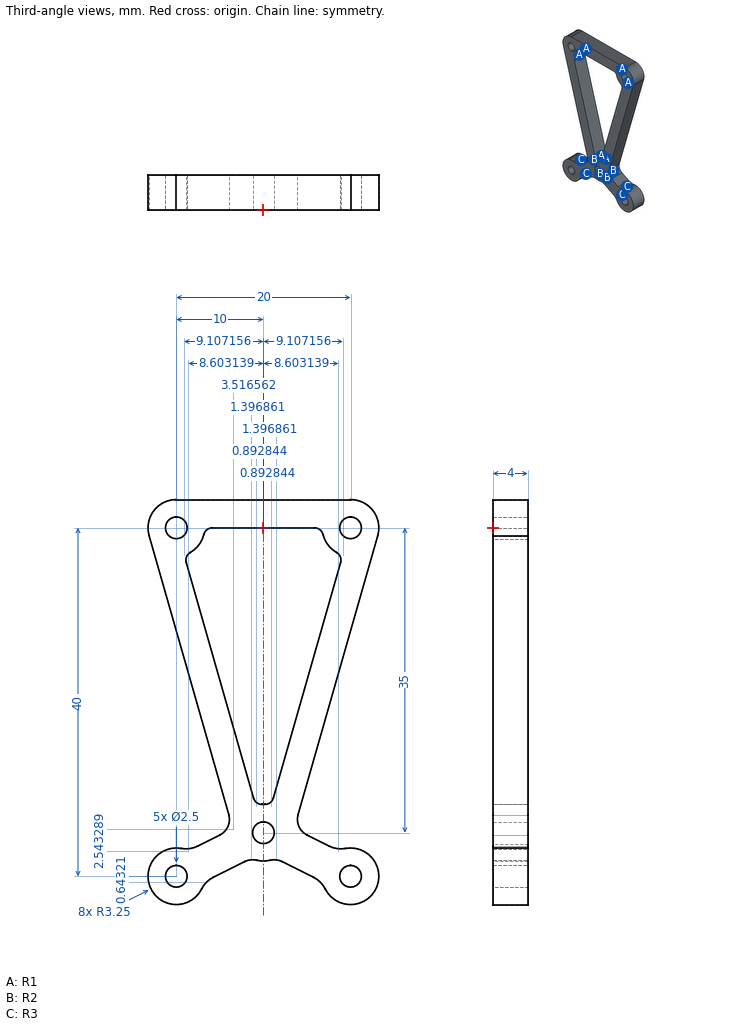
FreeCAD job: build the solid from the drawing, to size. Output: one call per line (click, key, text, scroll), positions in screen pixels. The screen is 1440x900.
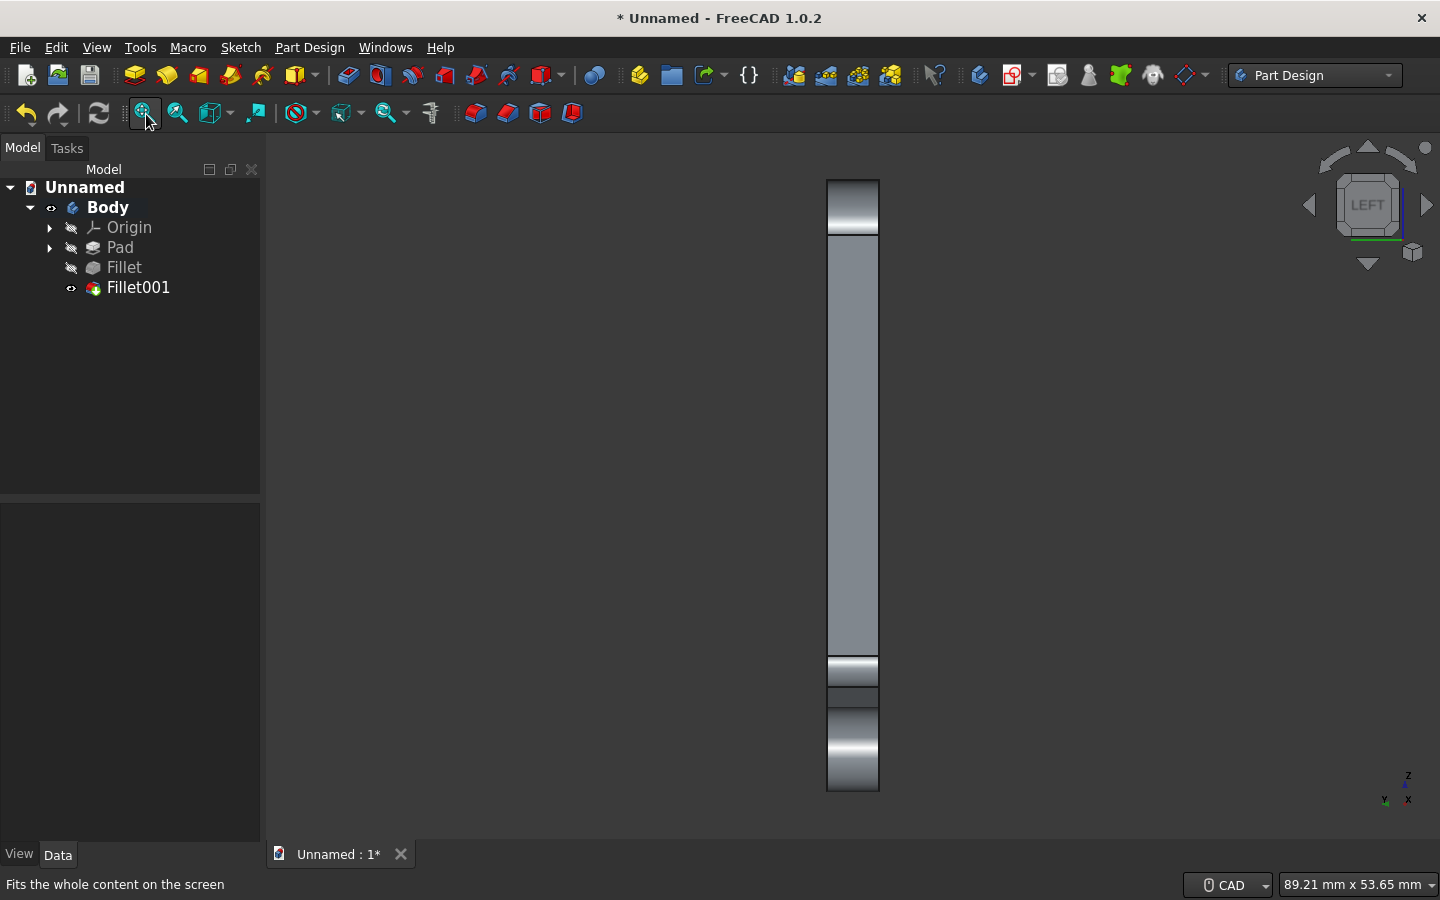
key(v)
key(3)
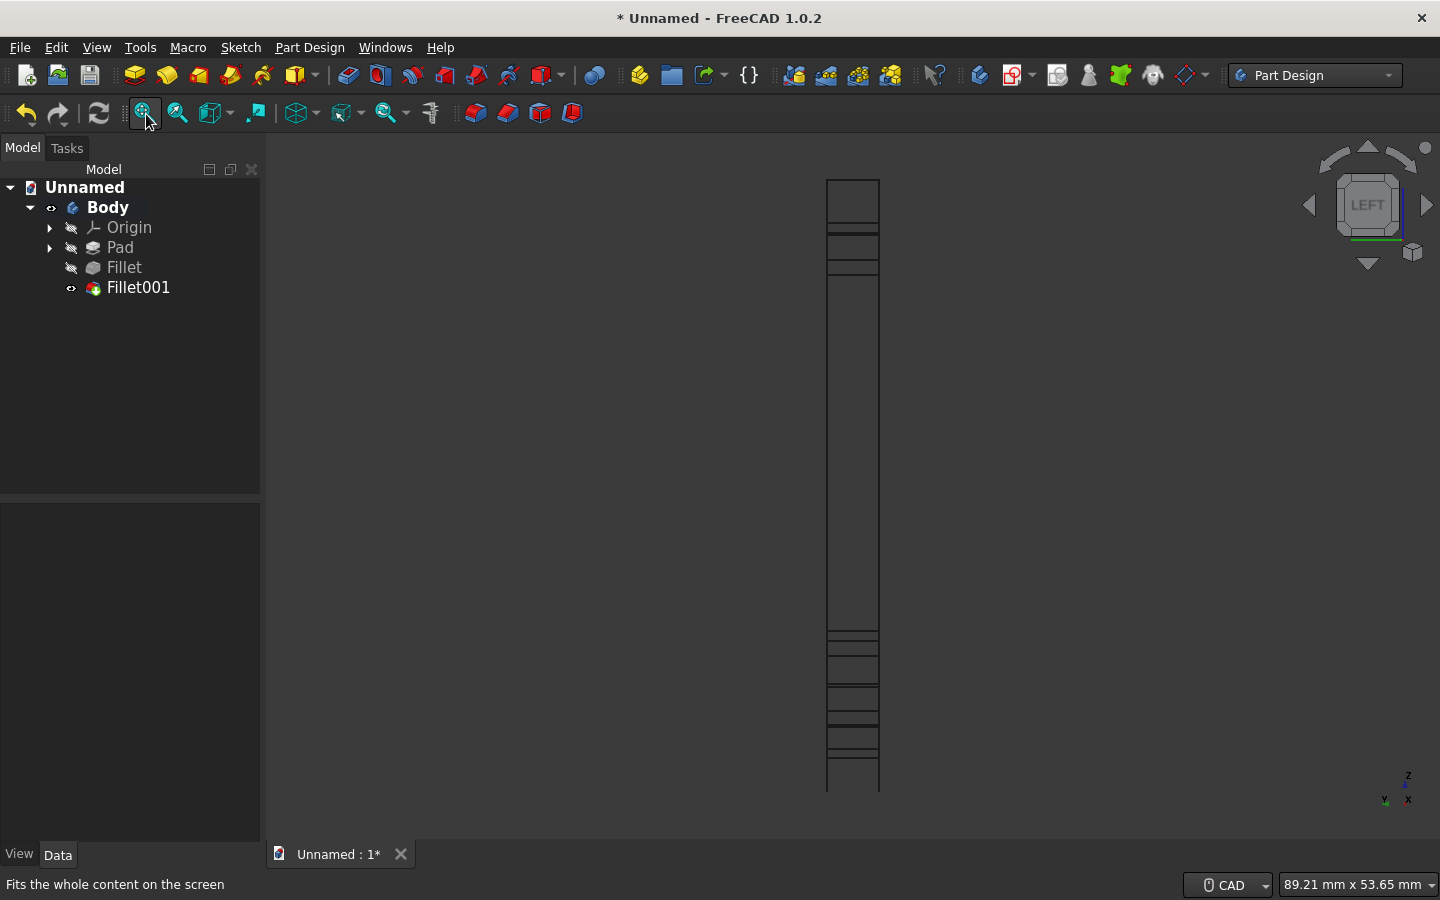
key(0)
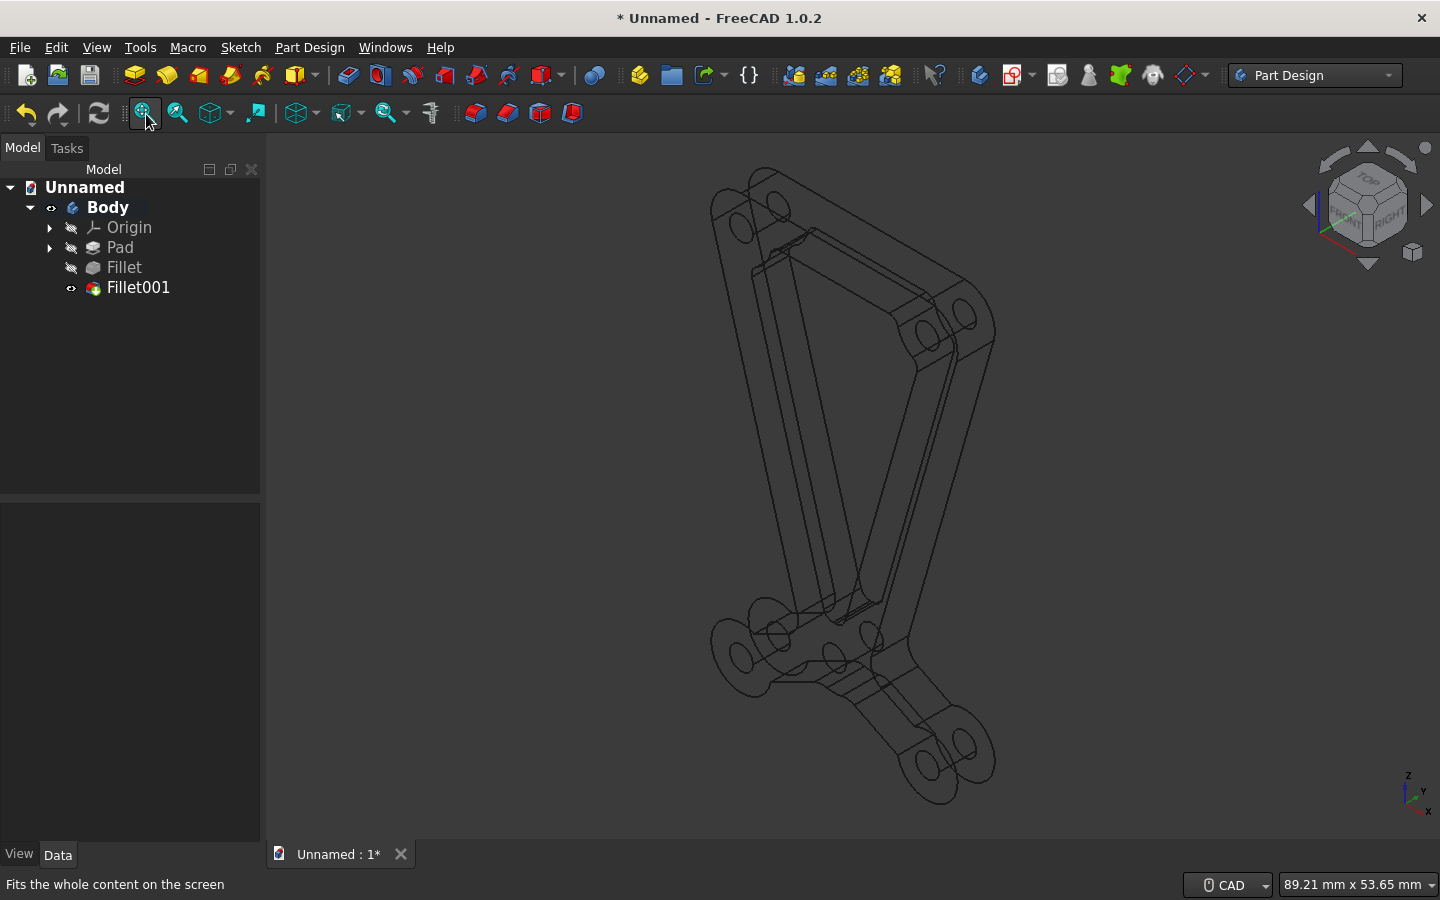
click(773, 622)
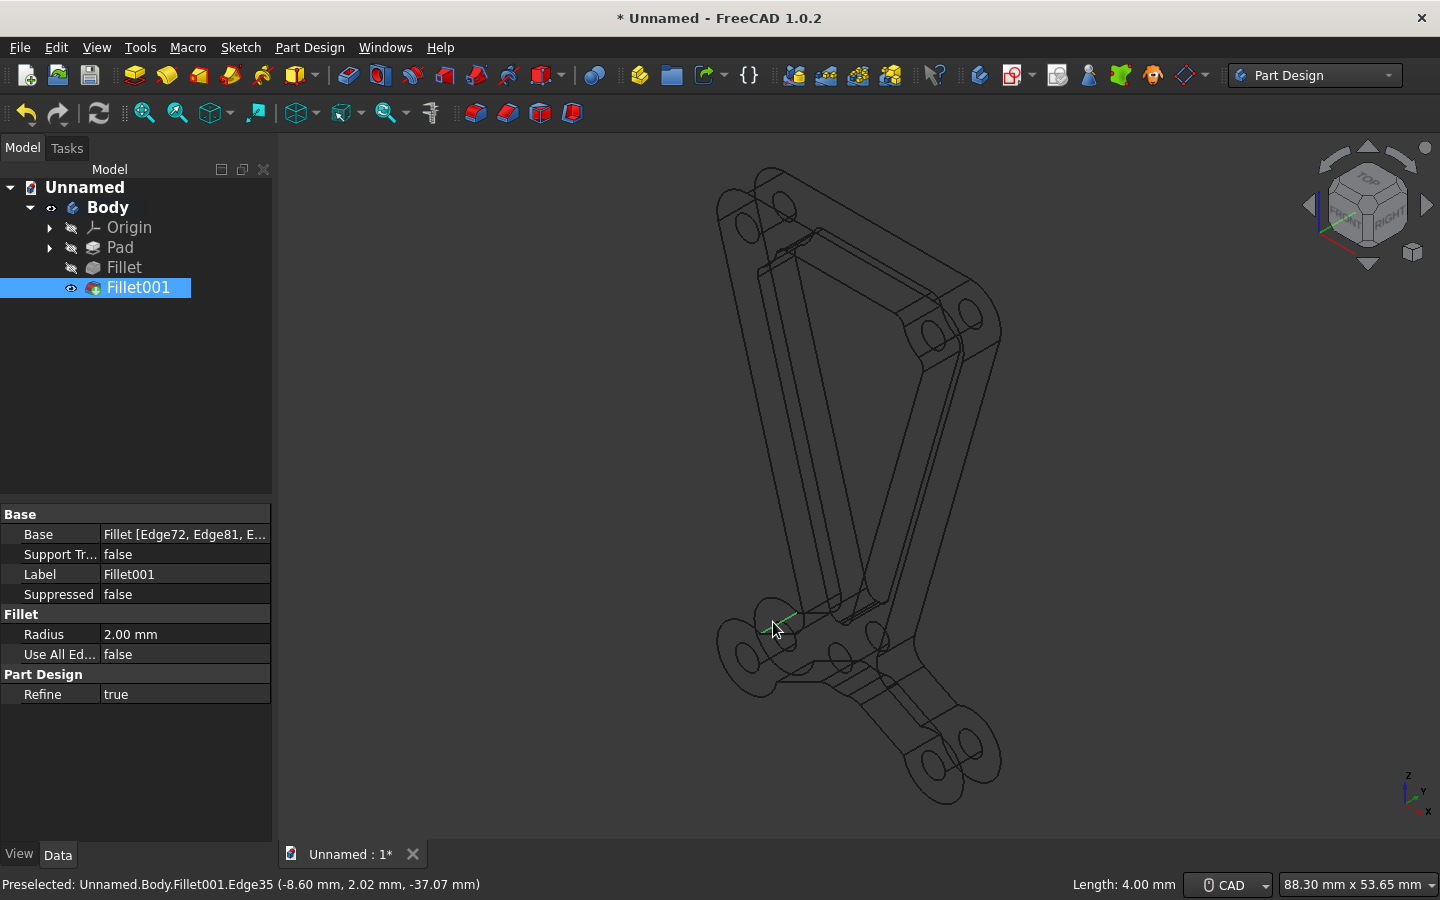
click(796, 670, ctrl)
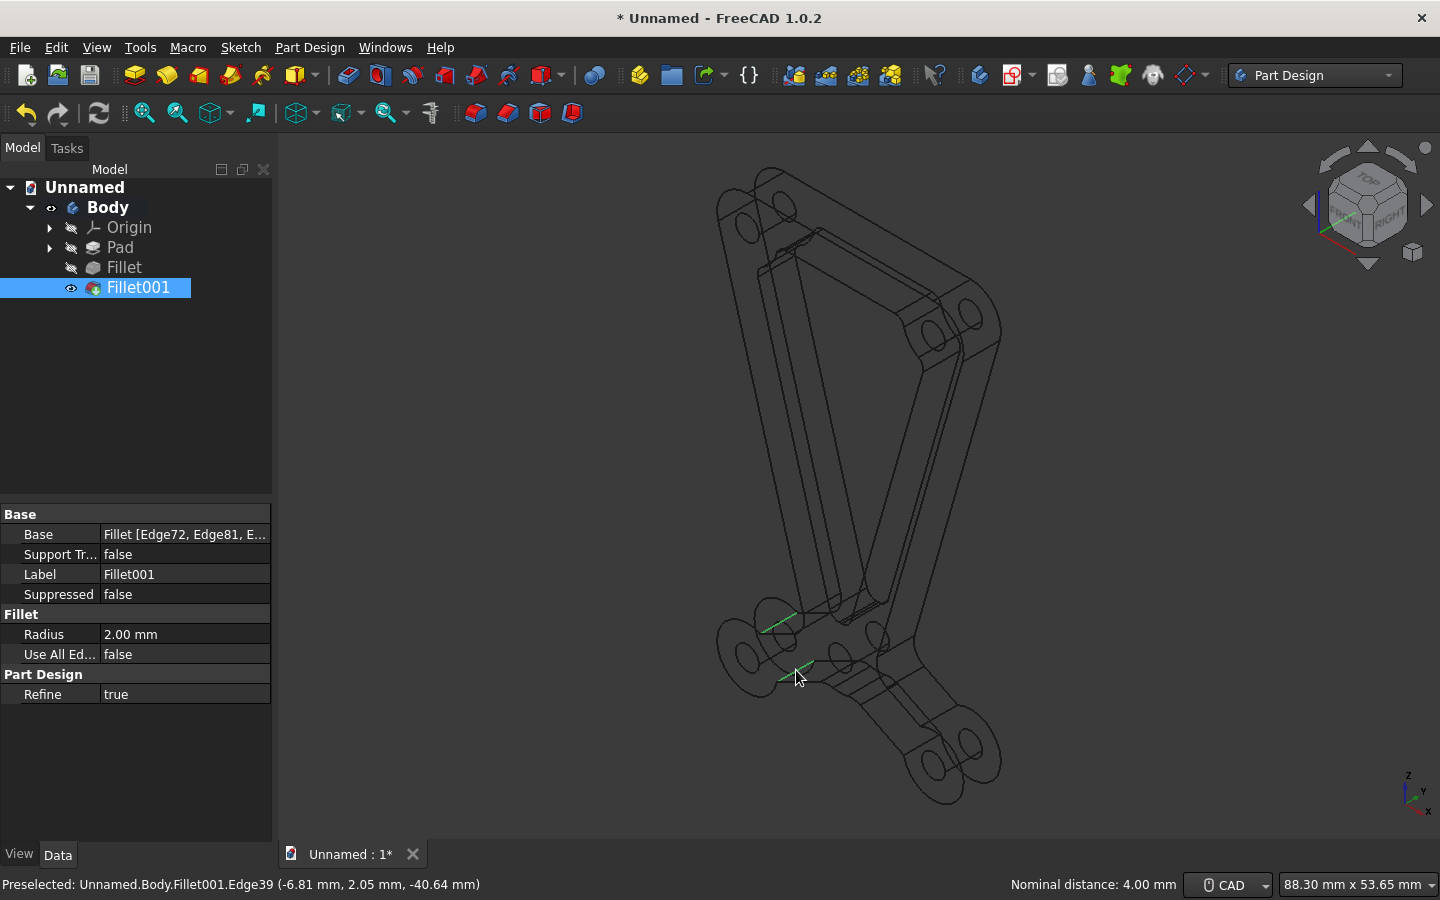
click(922, 744, ctrl)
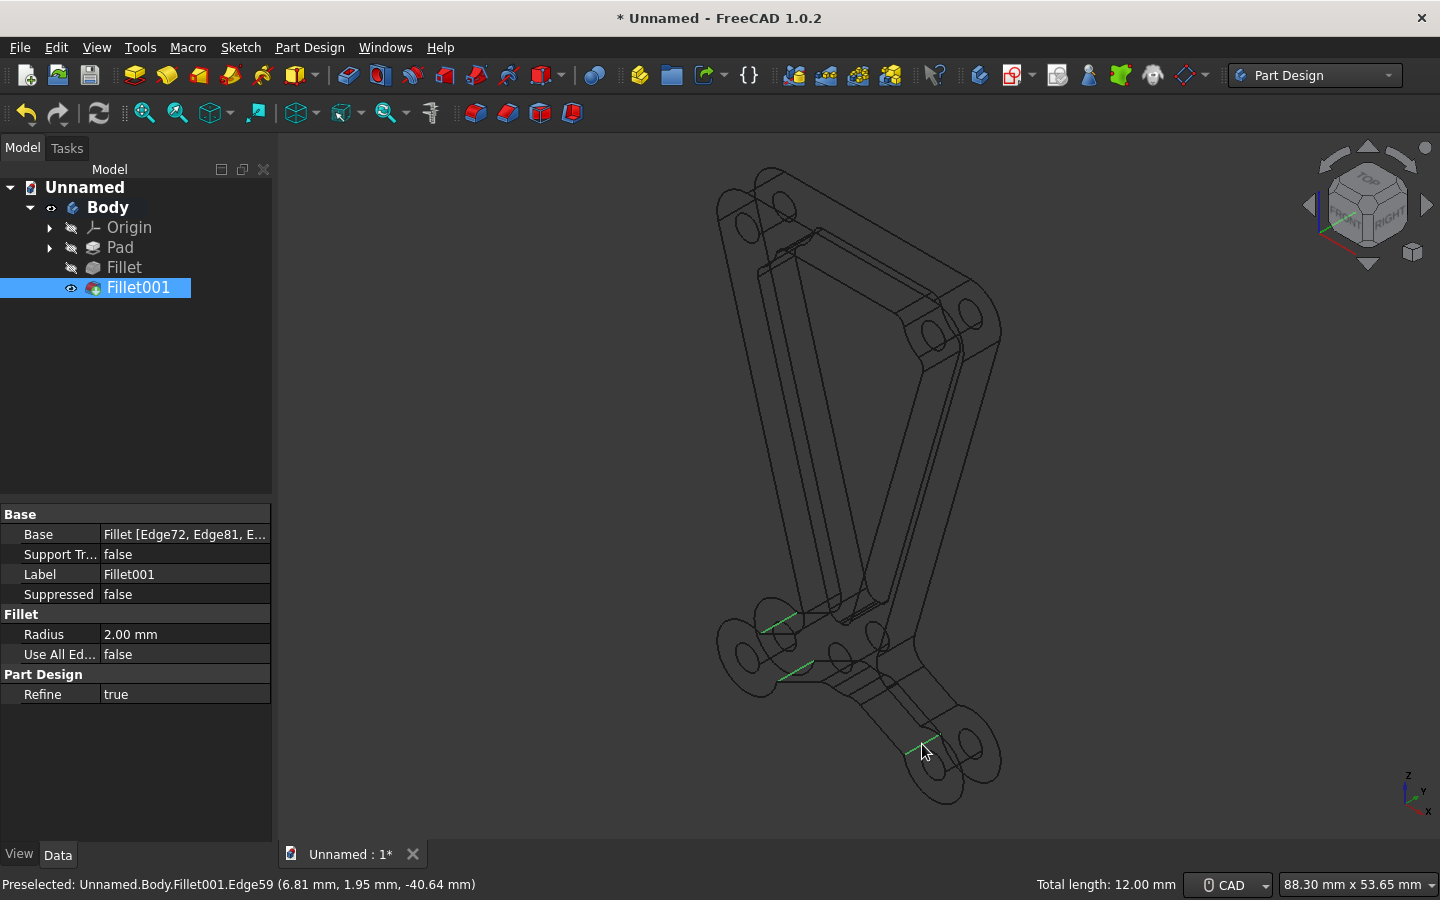
click(939, 715, ctrl)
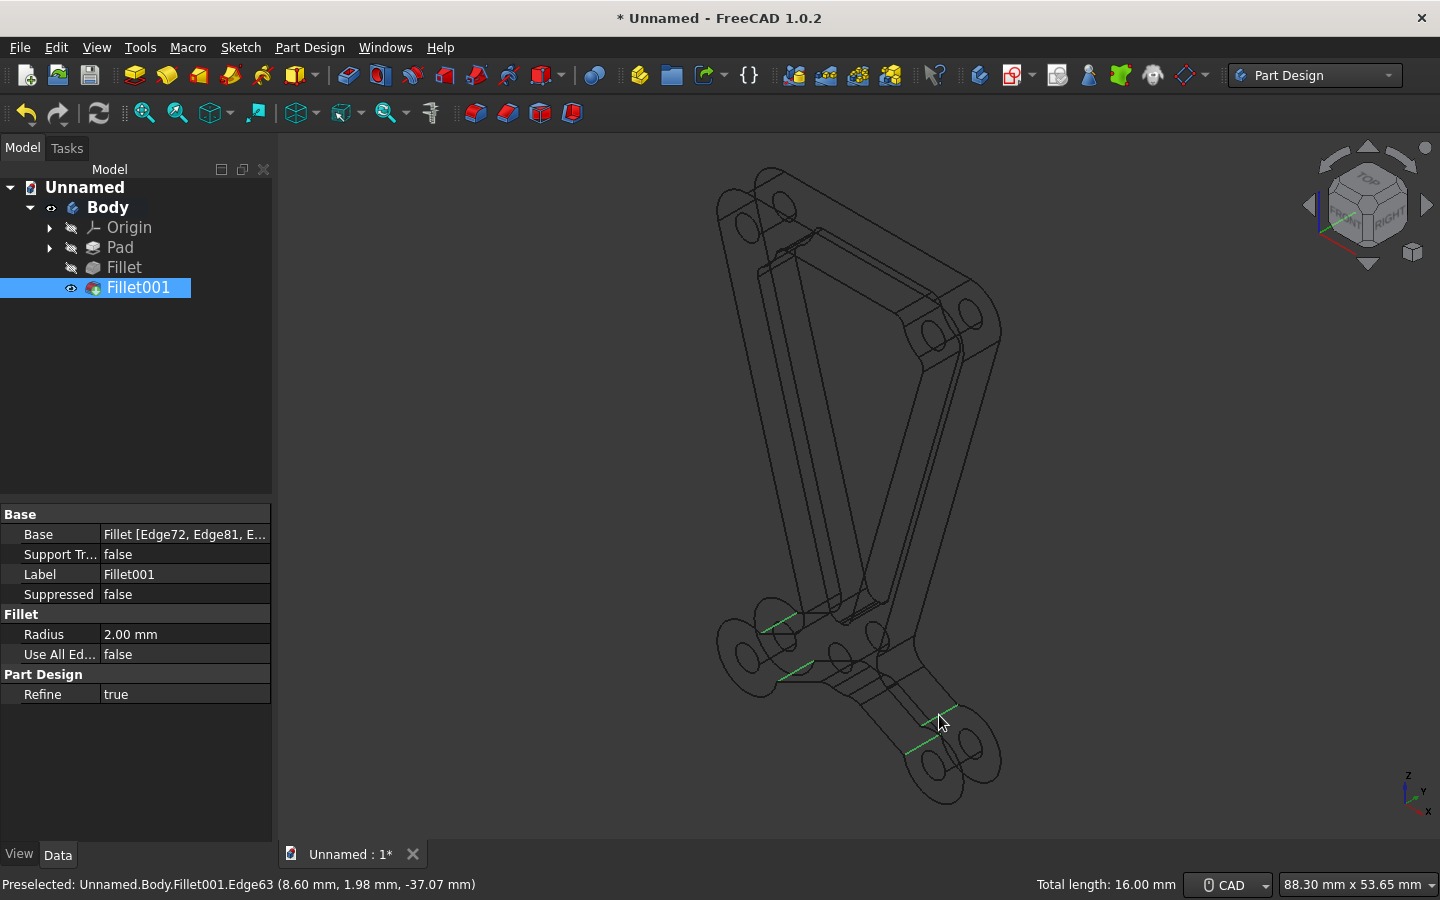
key(v)
key(1)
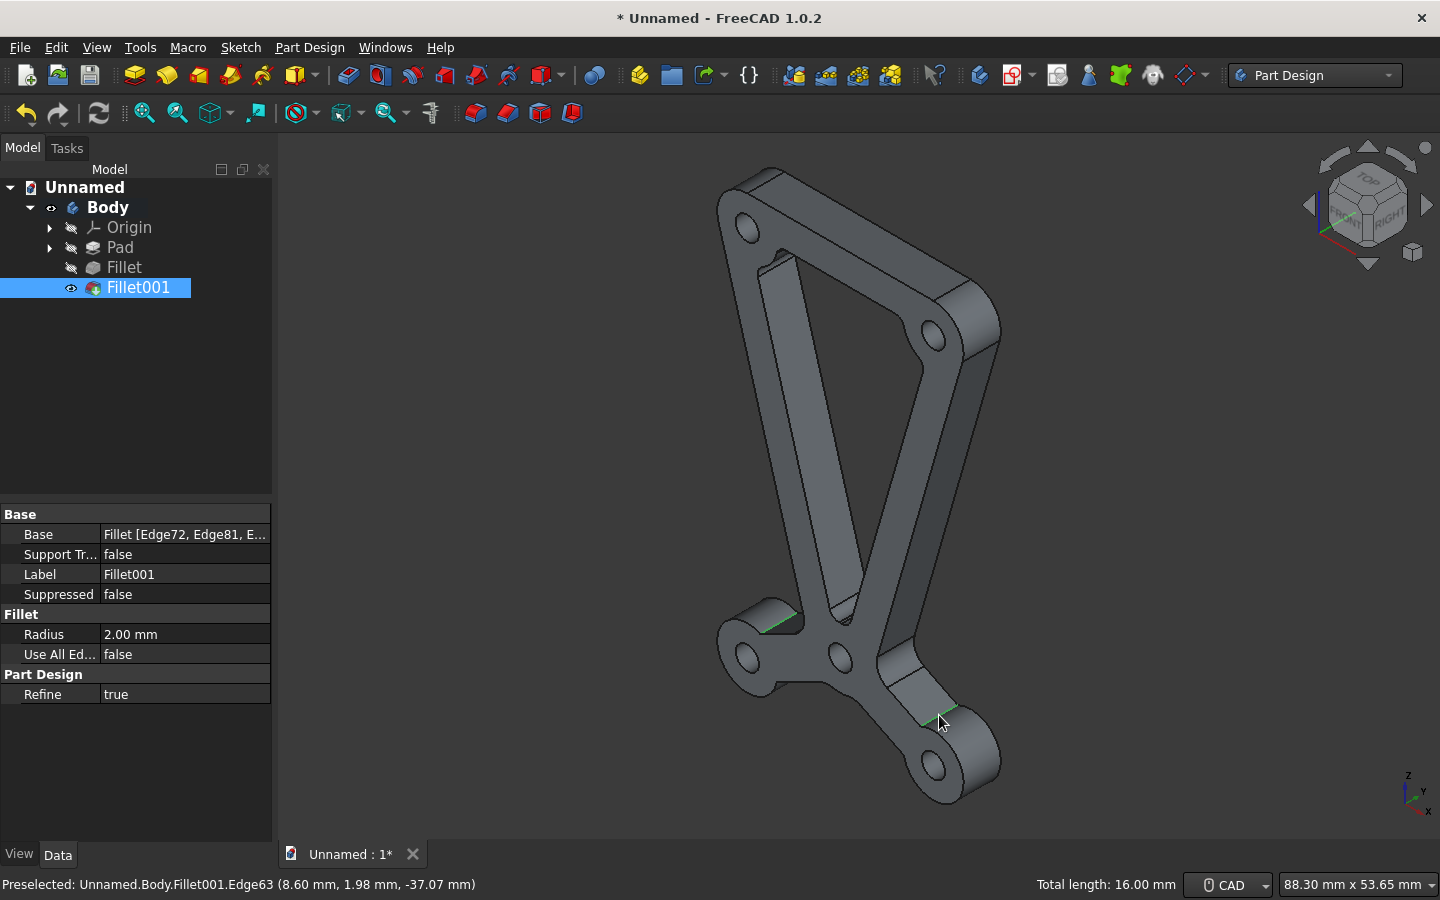
click(476, 114)